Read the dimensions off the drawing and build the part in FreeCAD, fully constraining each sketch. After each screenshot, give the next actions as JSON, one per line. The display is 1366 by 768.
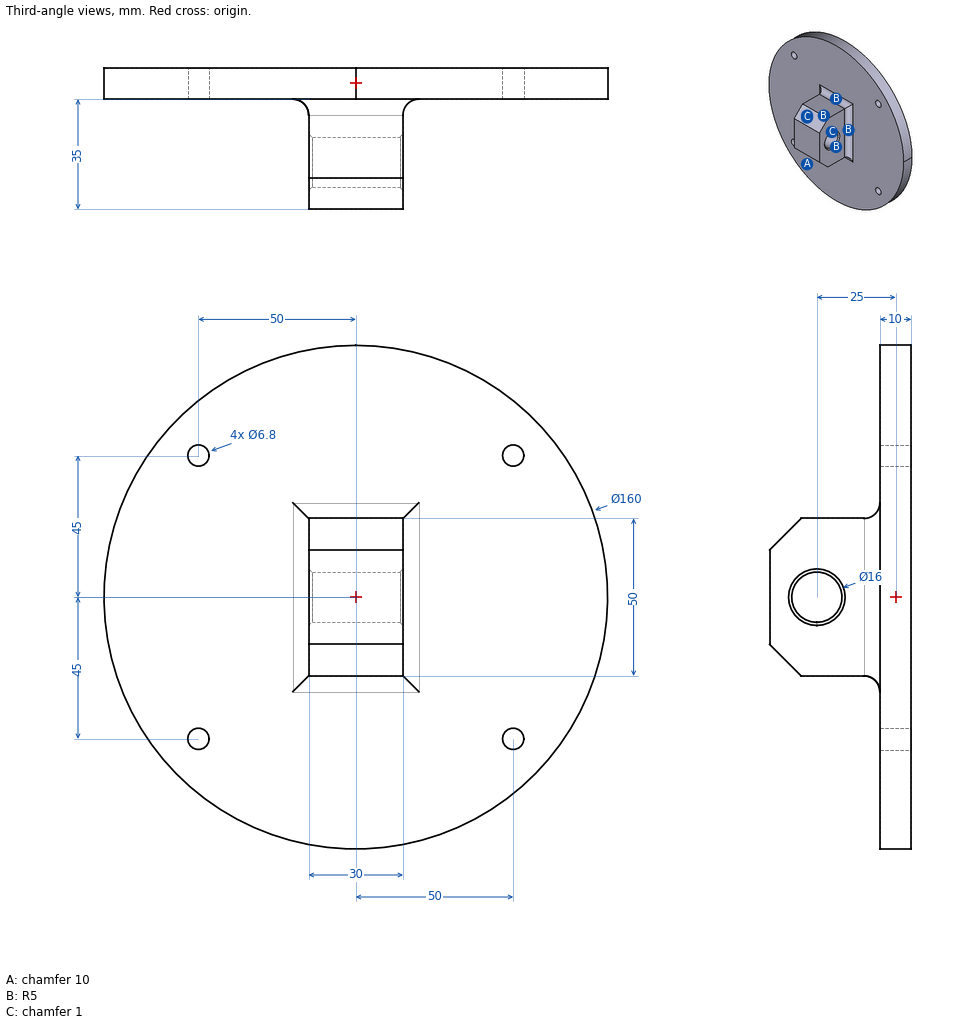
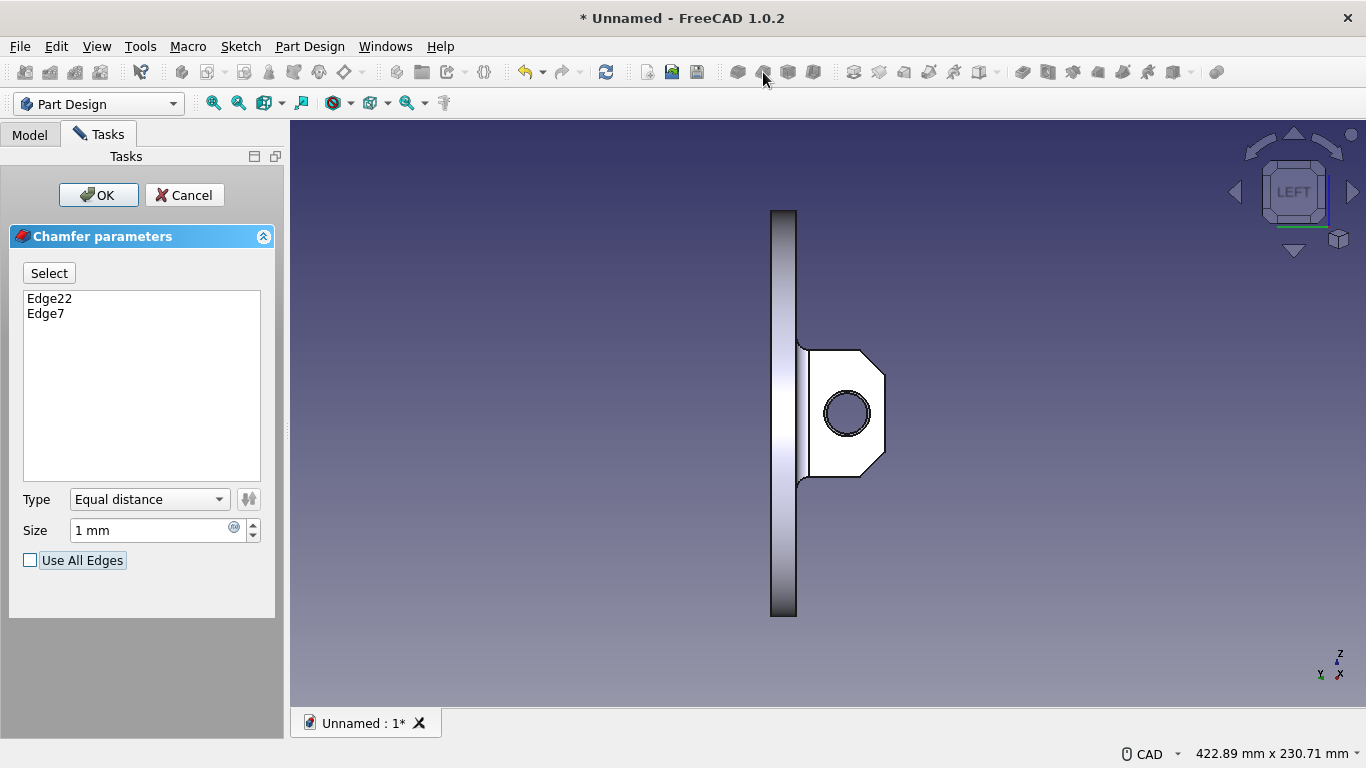
{"action": "left_click", "coordinate": [99, 195]}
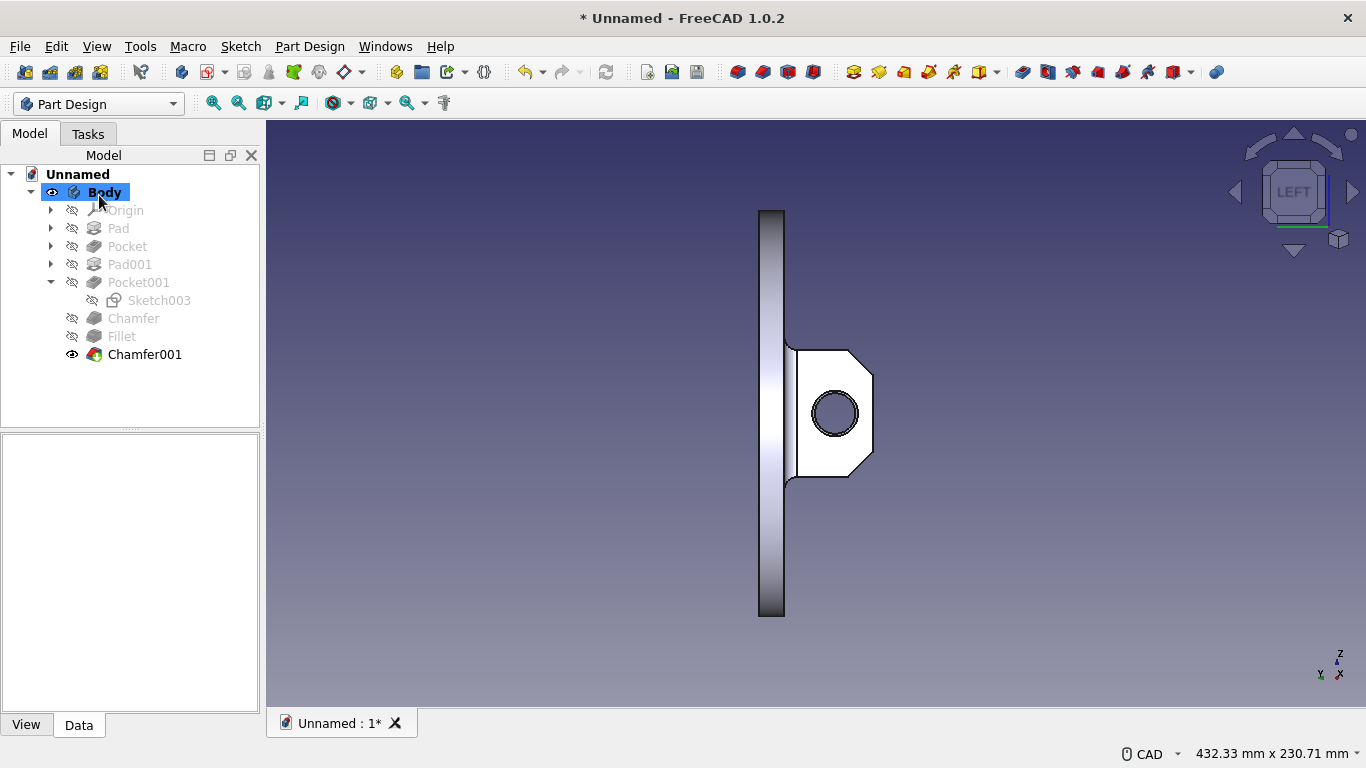
{"action": "key", "text": "0"}